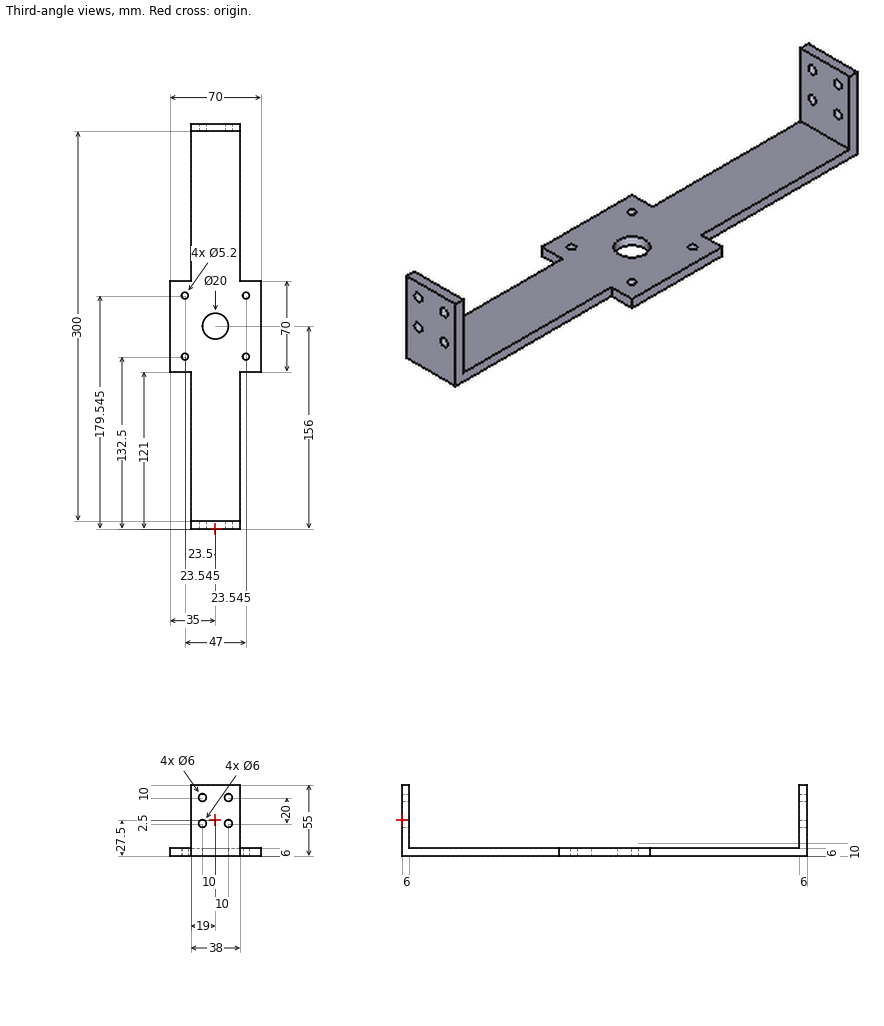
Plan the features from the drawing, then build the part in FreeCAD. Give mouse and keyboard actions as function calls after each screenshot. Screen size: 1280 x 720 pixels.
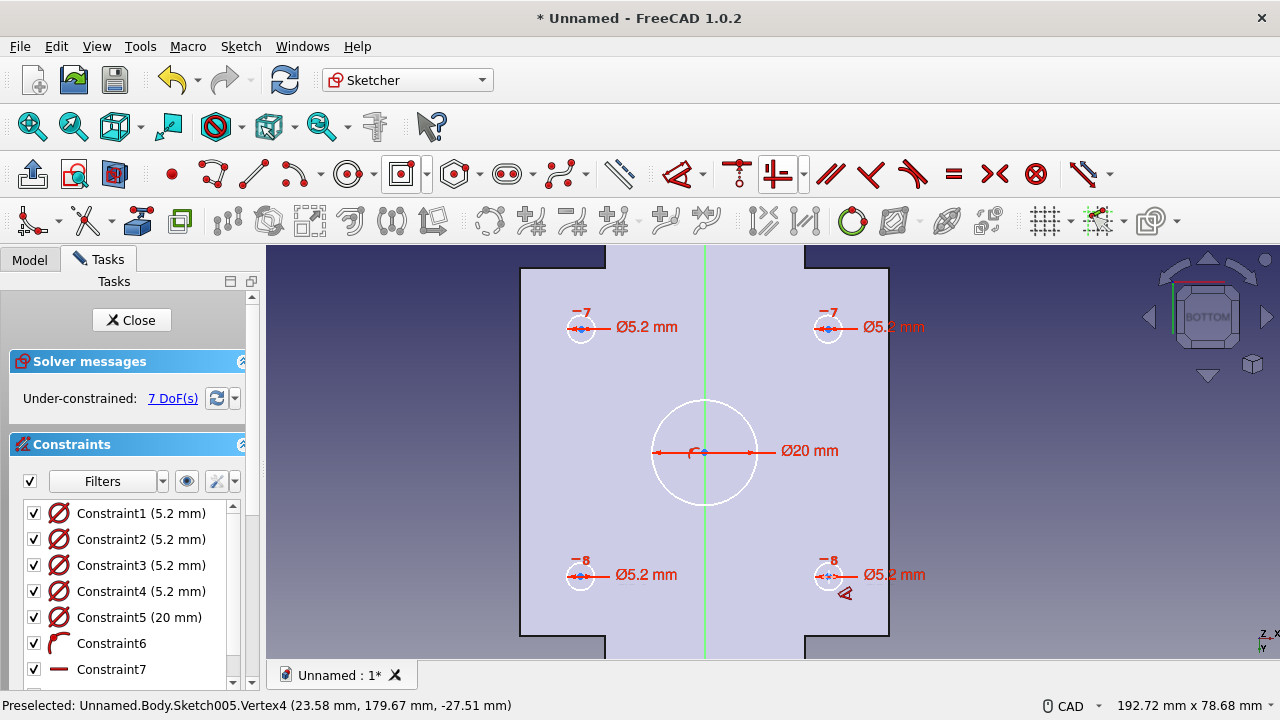
click(705, 453)
click(739, 363)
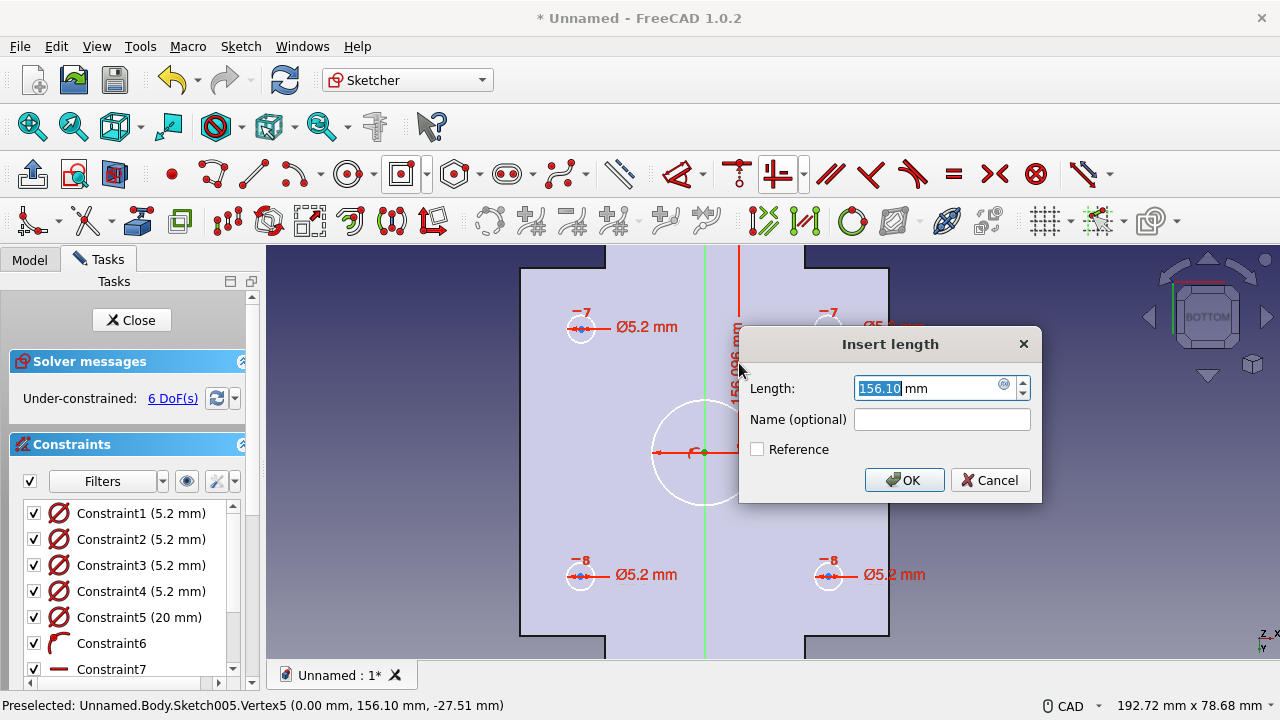
text(156)
key(Return)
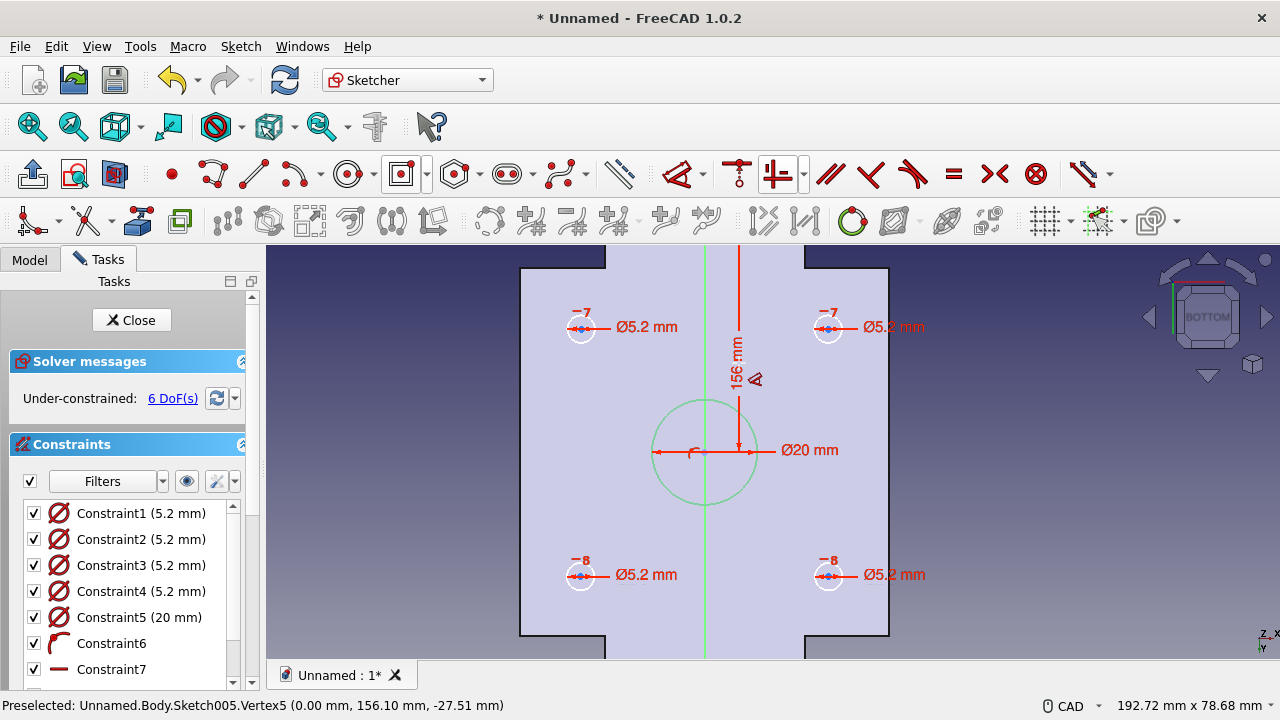
click(581, 329)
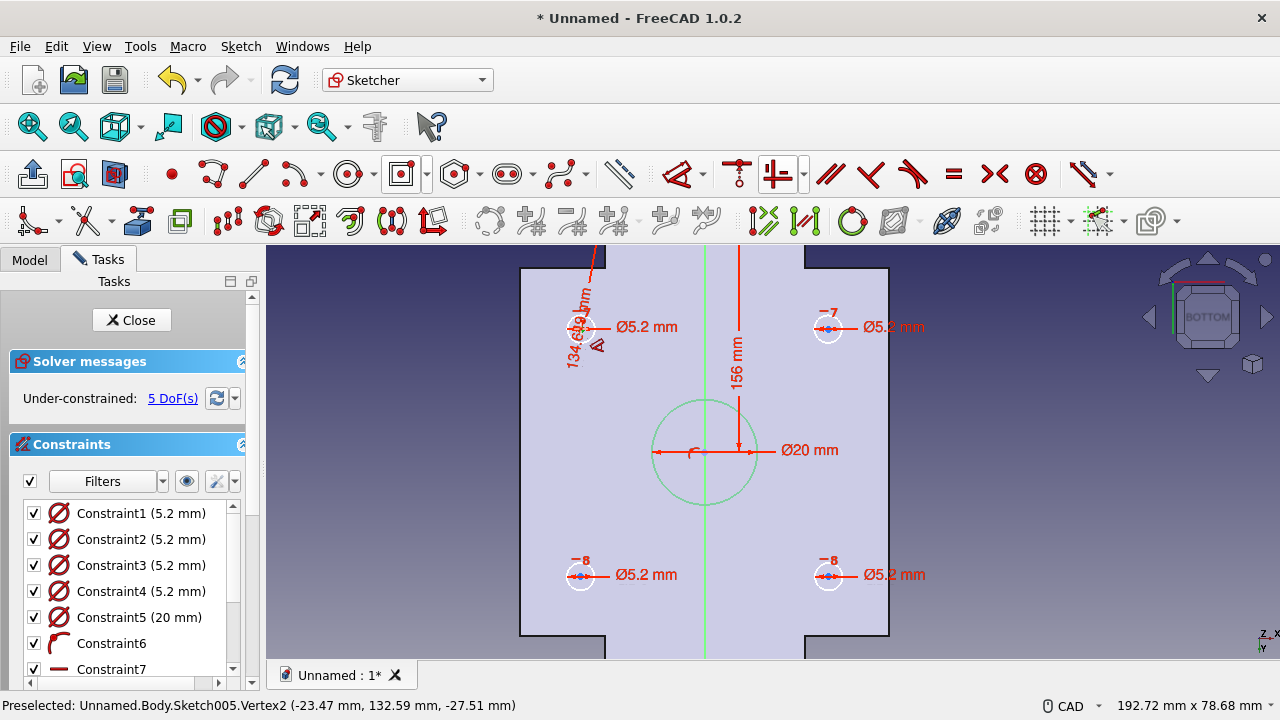
click(828, 329)
click(648, 295)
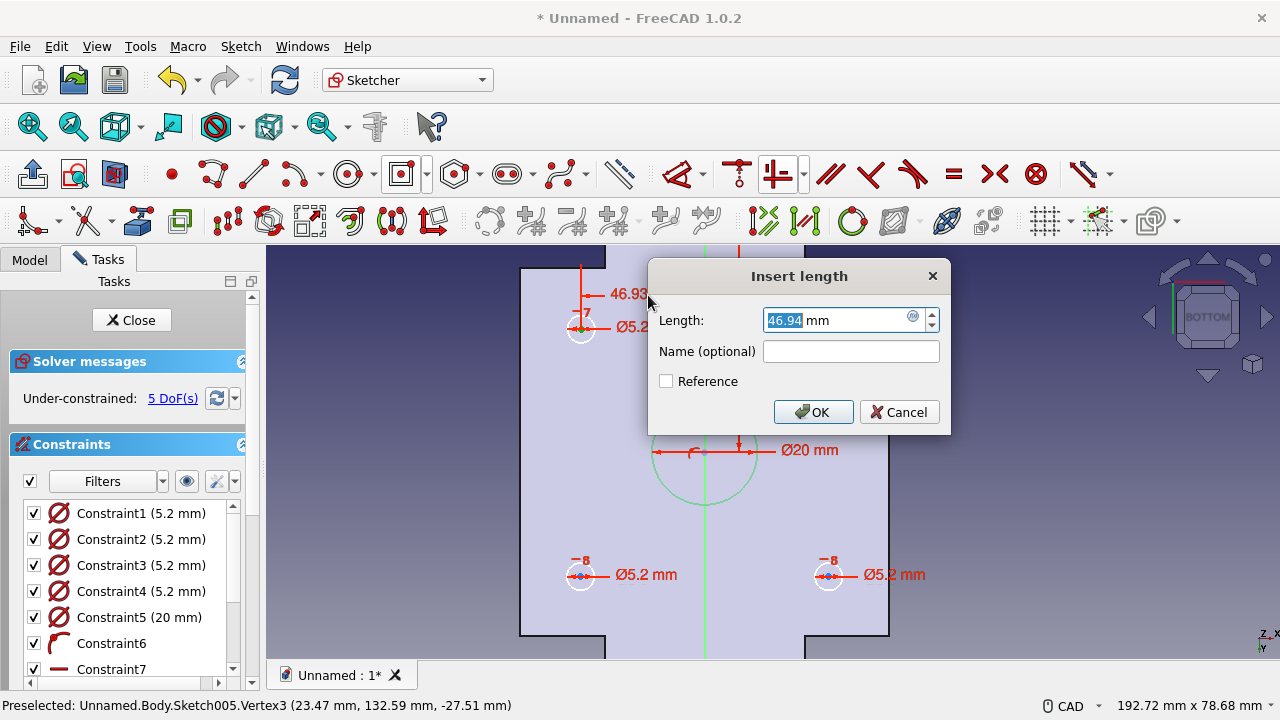
text(47)
key(Return)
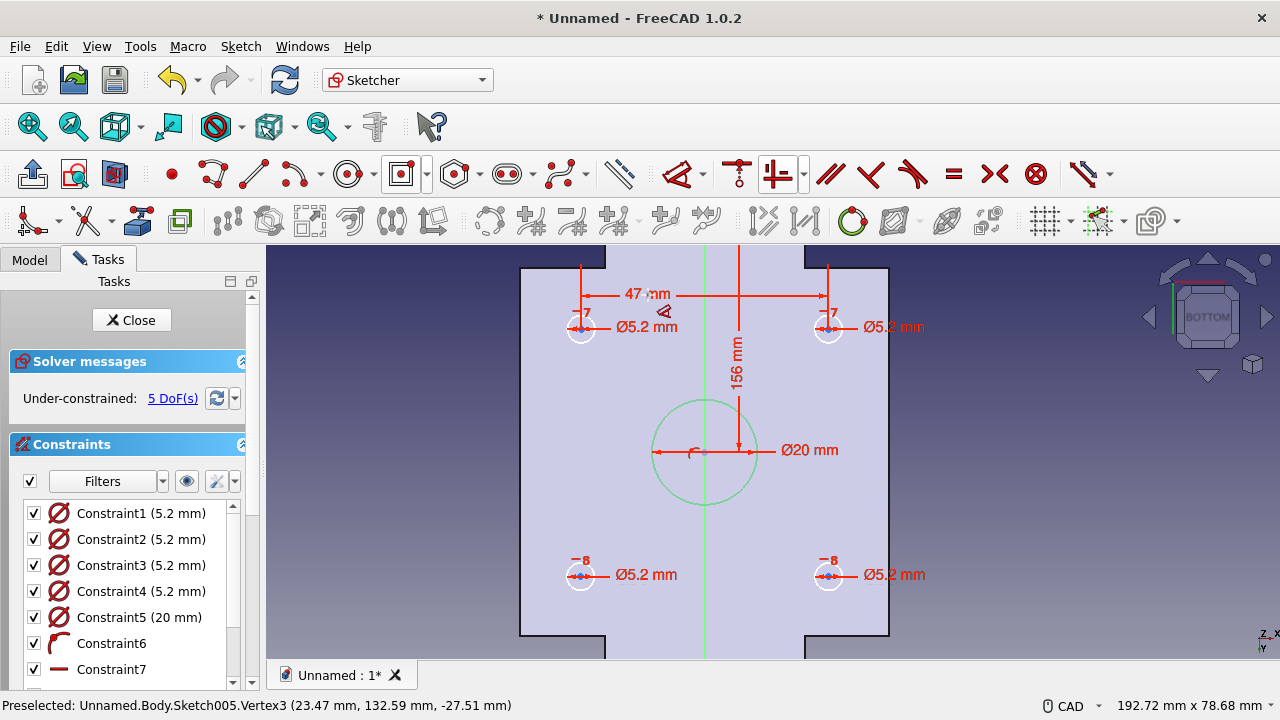
click(581, 329)
click(643, 363)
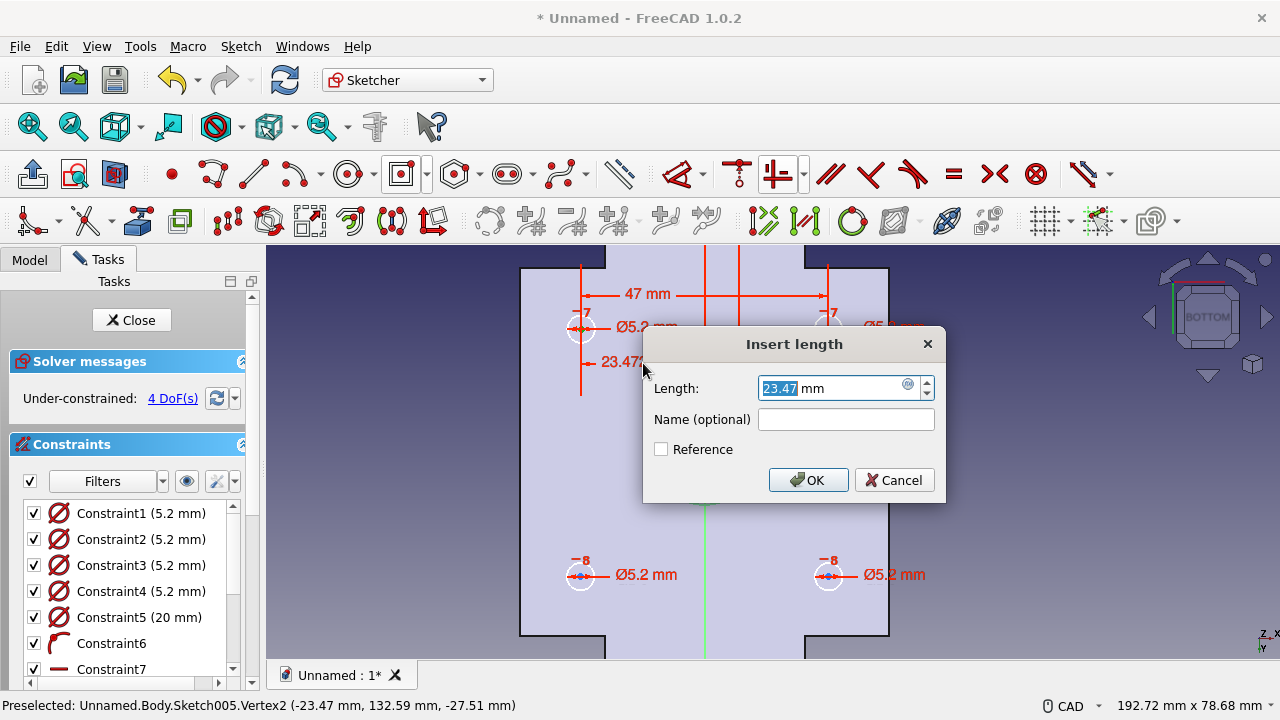
text(23.5)
key(Return)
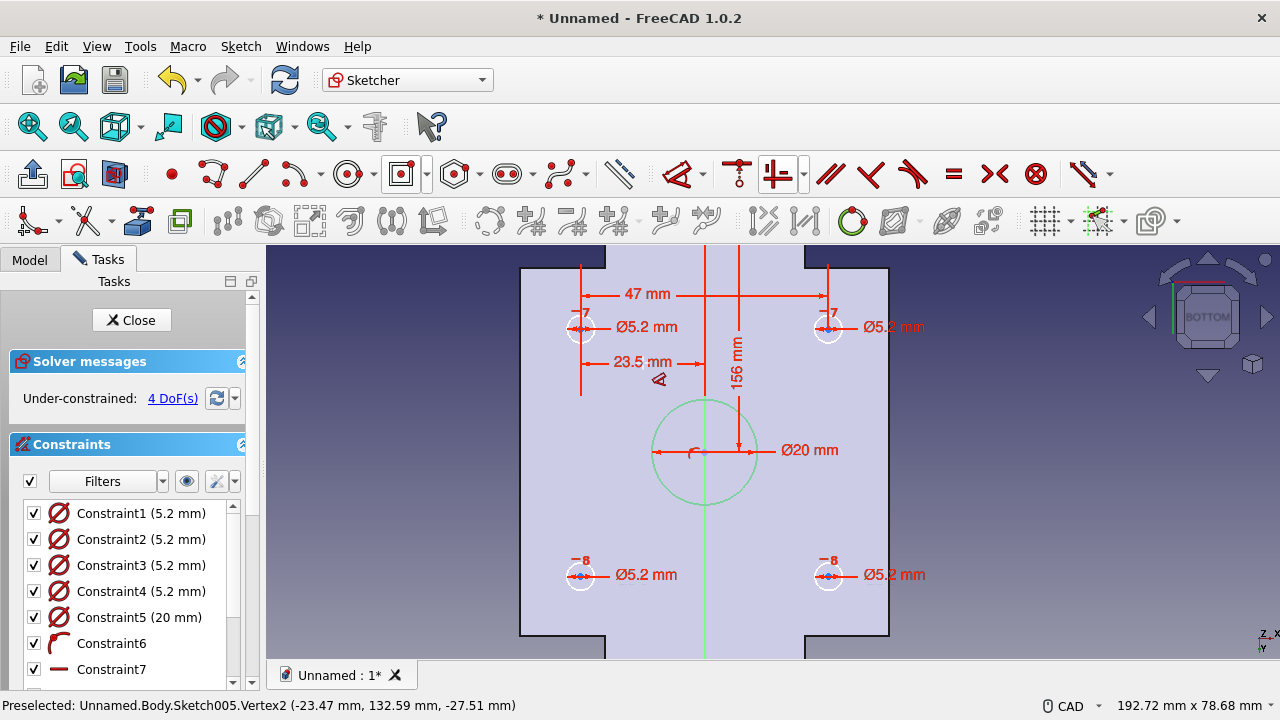
click(581, 329)
click(547, 301)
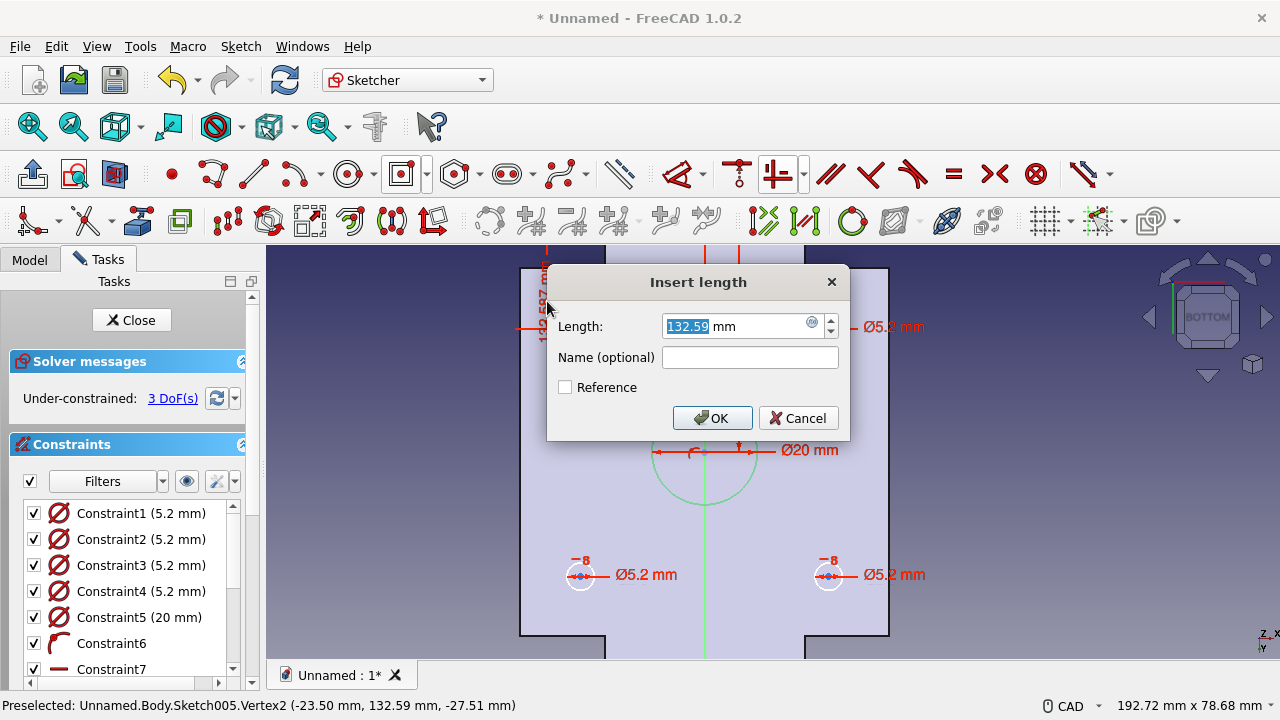
text(132.5)
key(Return)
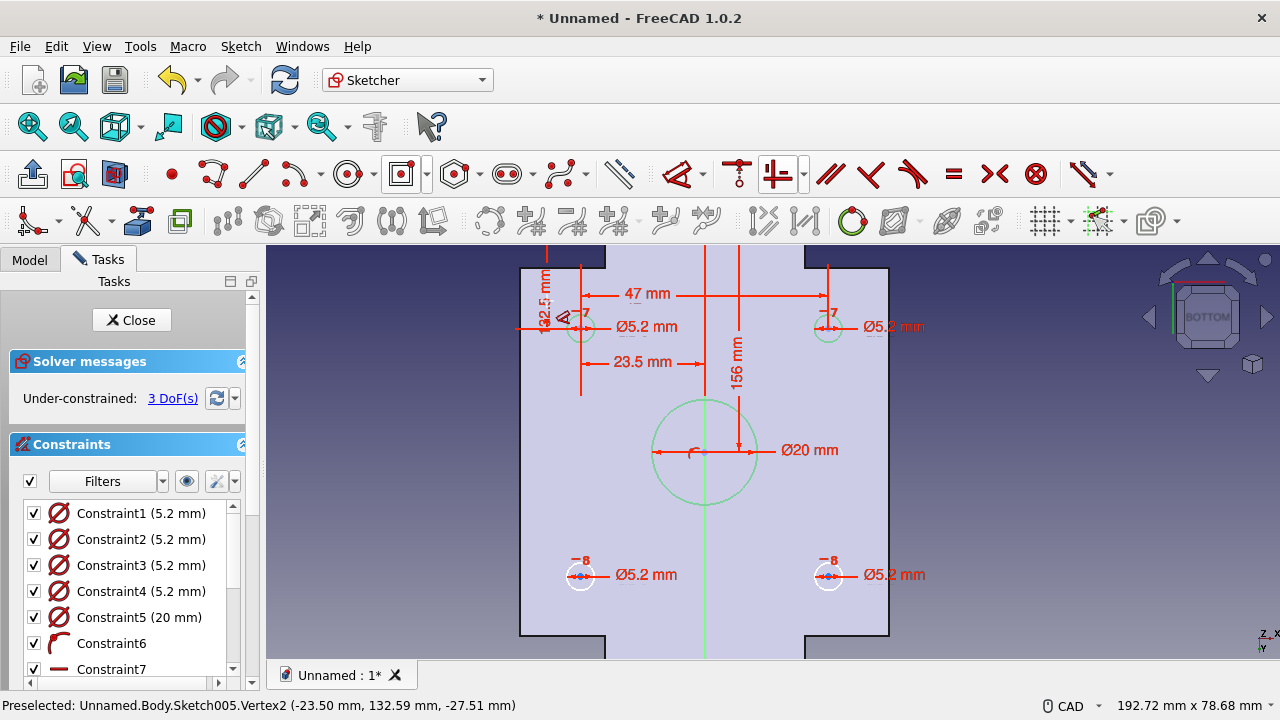
click(581, 577)
click(643, 611)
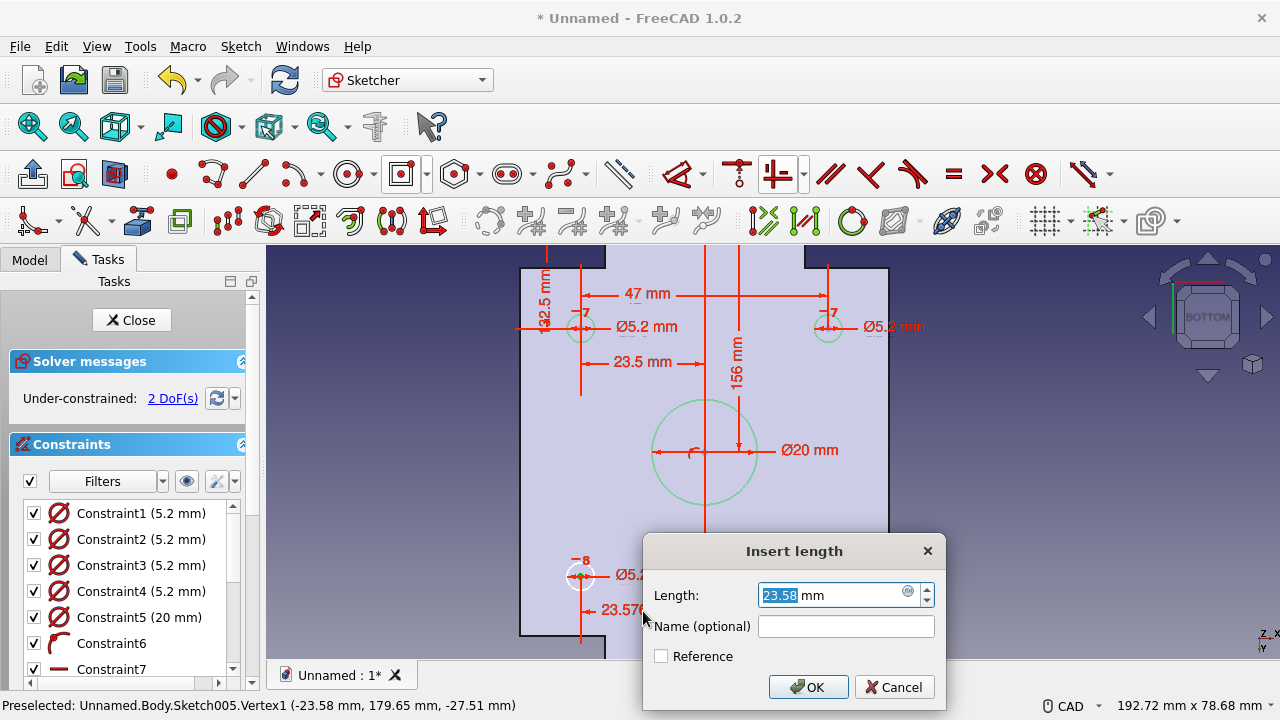
text(23.545)
key(Return)